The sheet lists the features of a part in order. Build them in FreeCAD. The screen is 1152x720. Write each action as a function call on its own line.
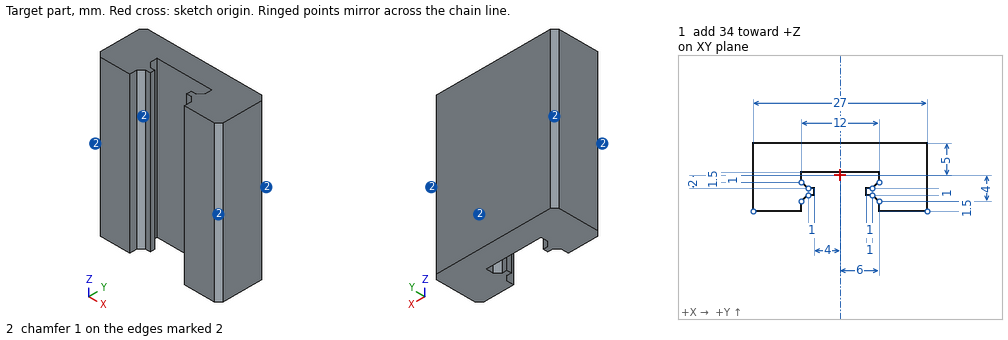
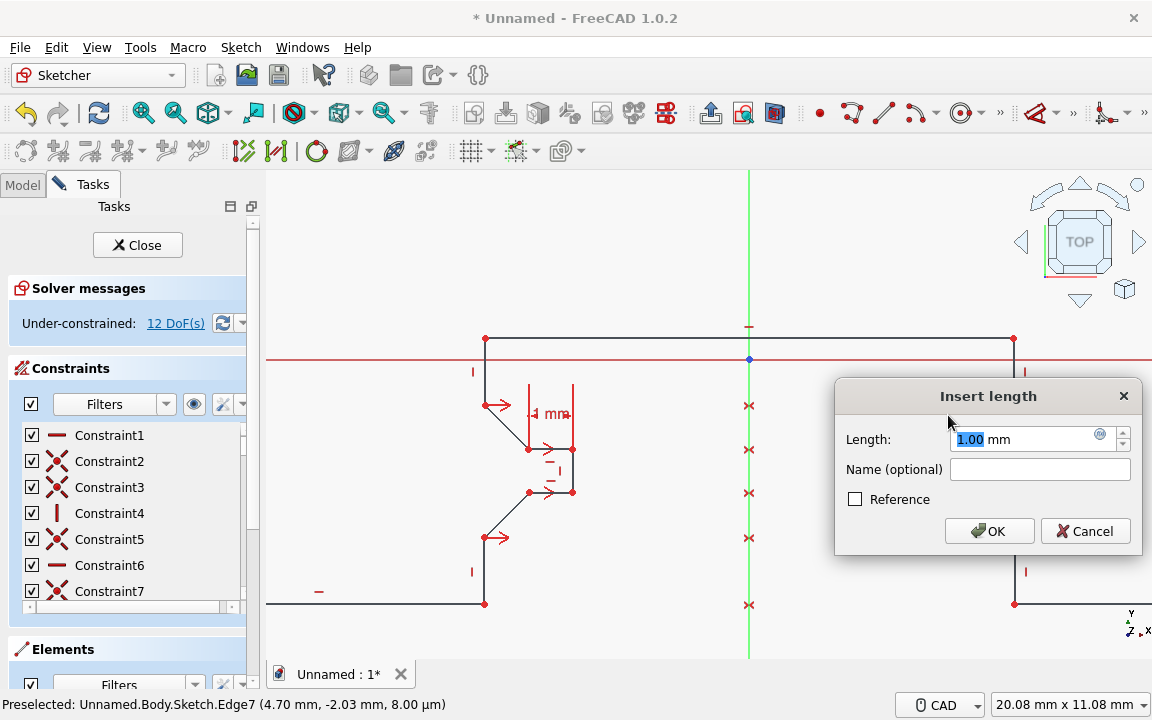
text(1)
key(Return)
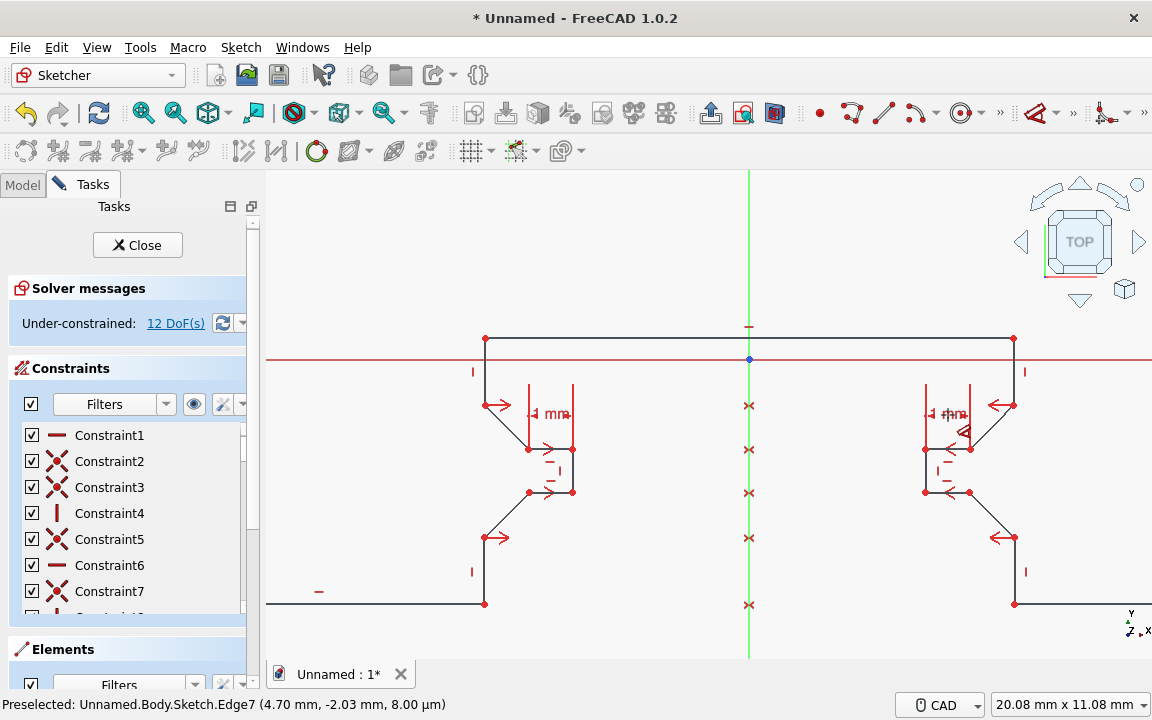
click(926, 462)
click(960, 471)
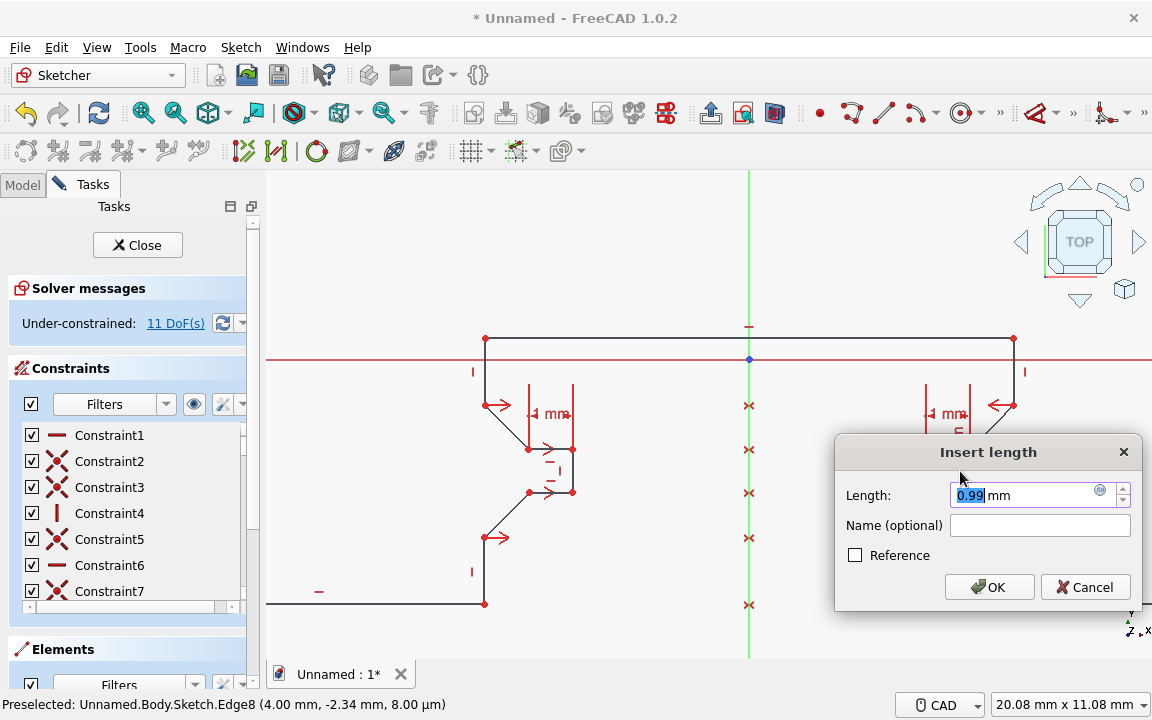
text(1)
key(Return)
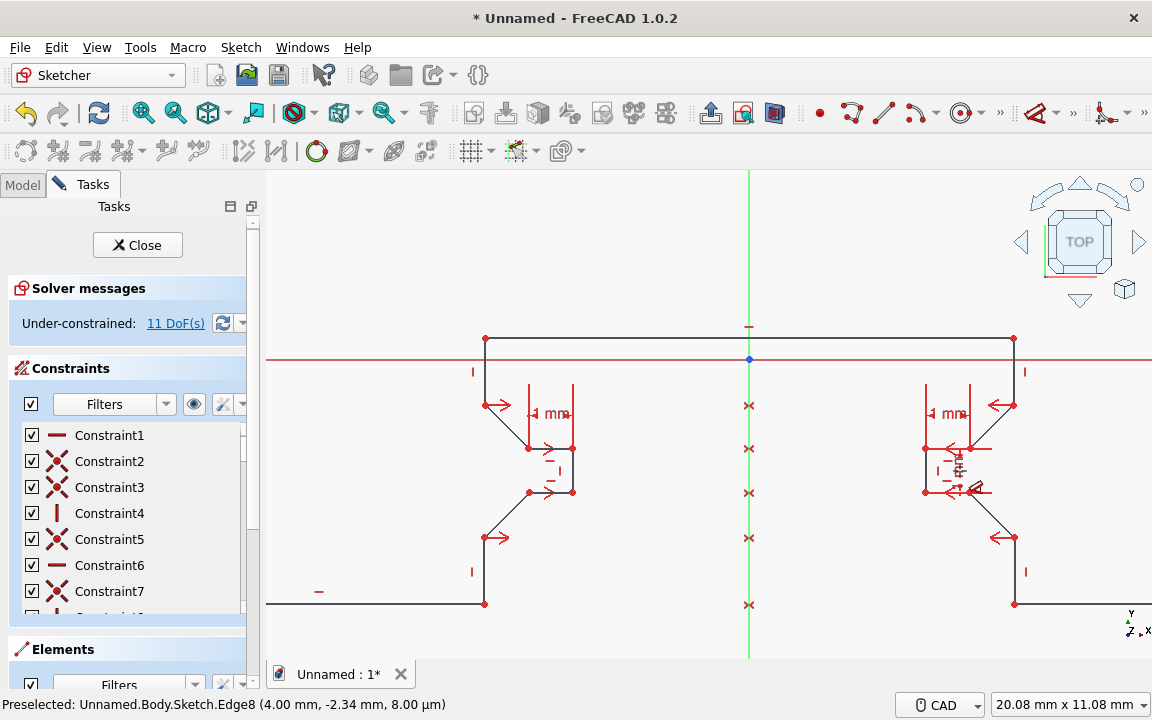
click(939, 493)
click(948, 527)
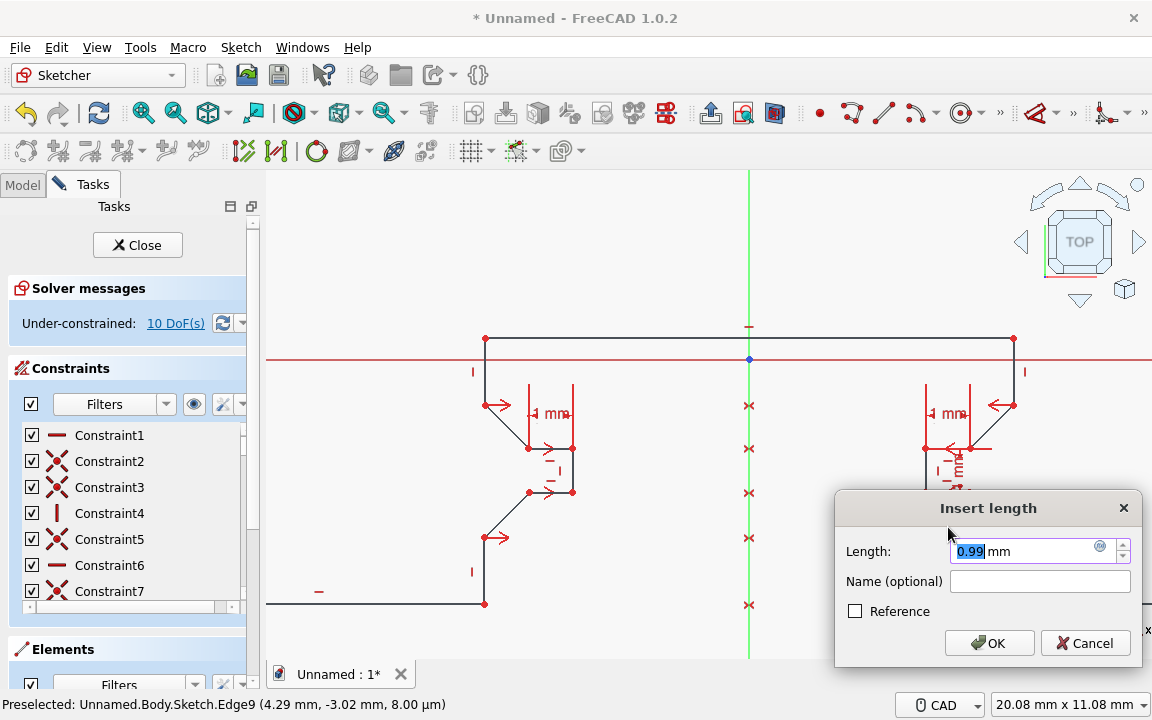
text(1)
key(Return)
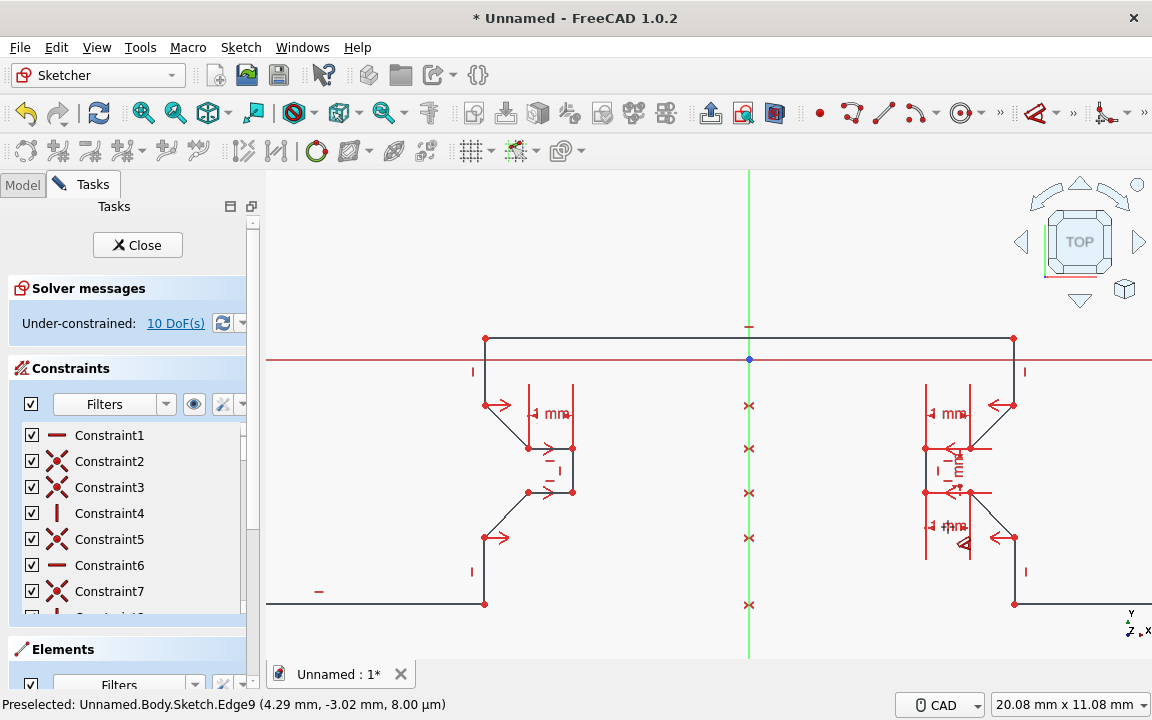
click(644, 338)
click(736, 304)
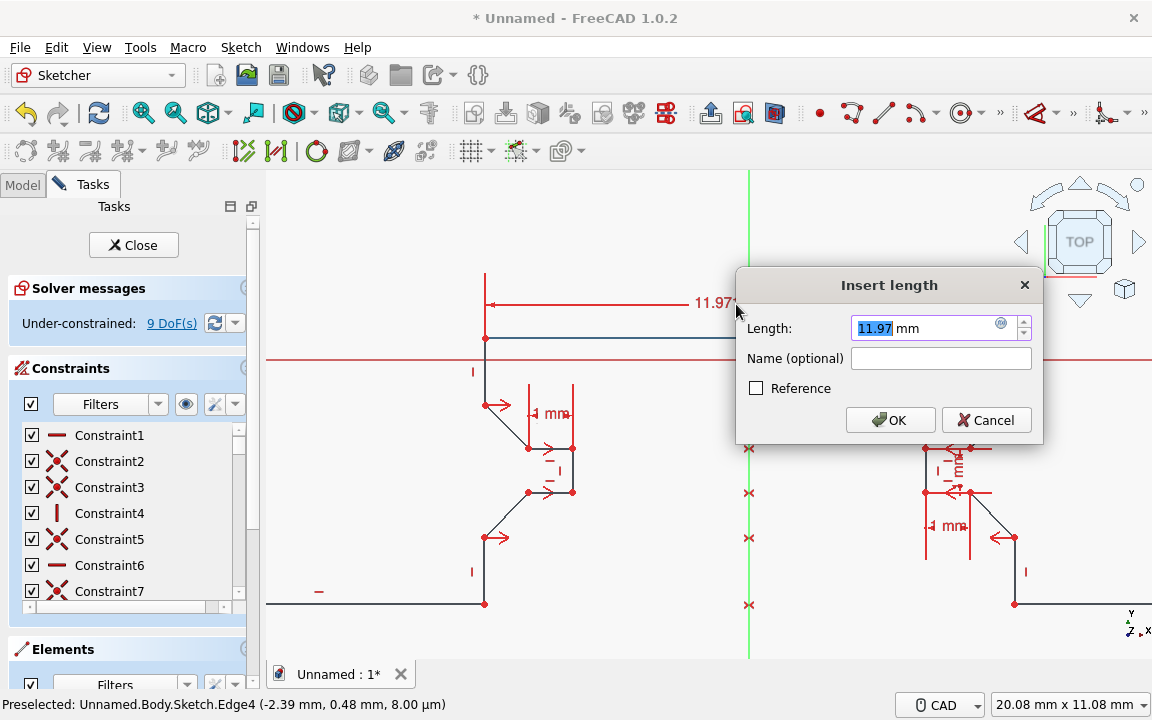
text(12)
key(Return)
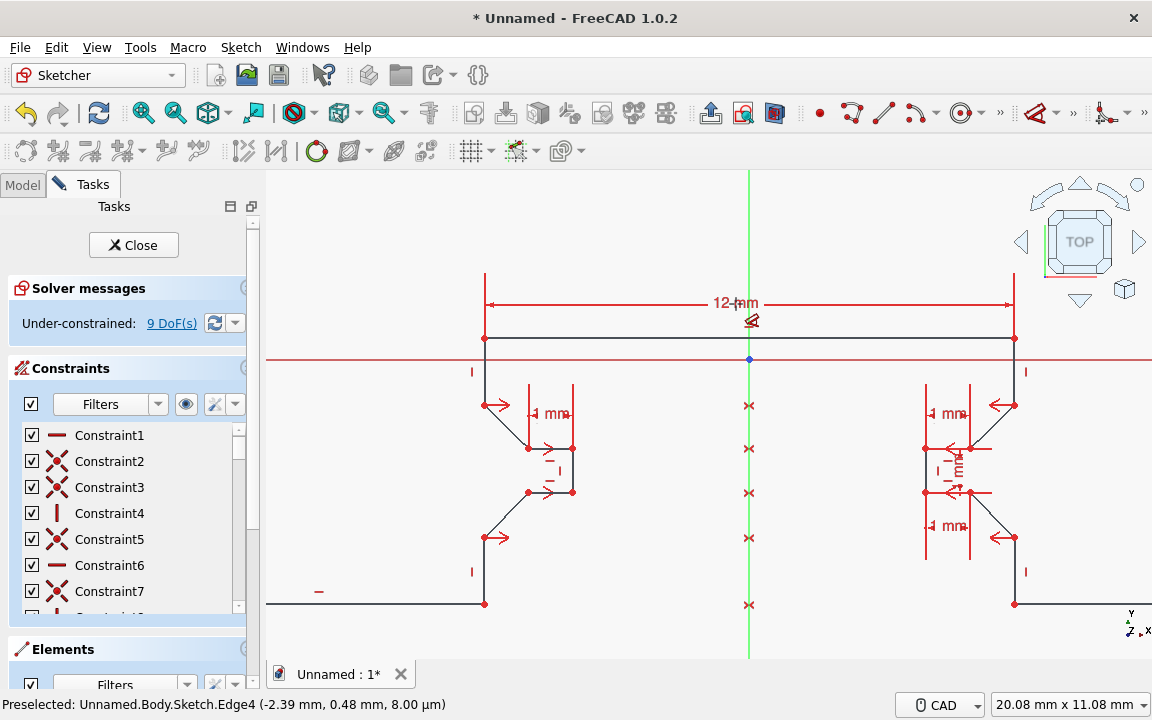
scroll(552, 450, down, 4)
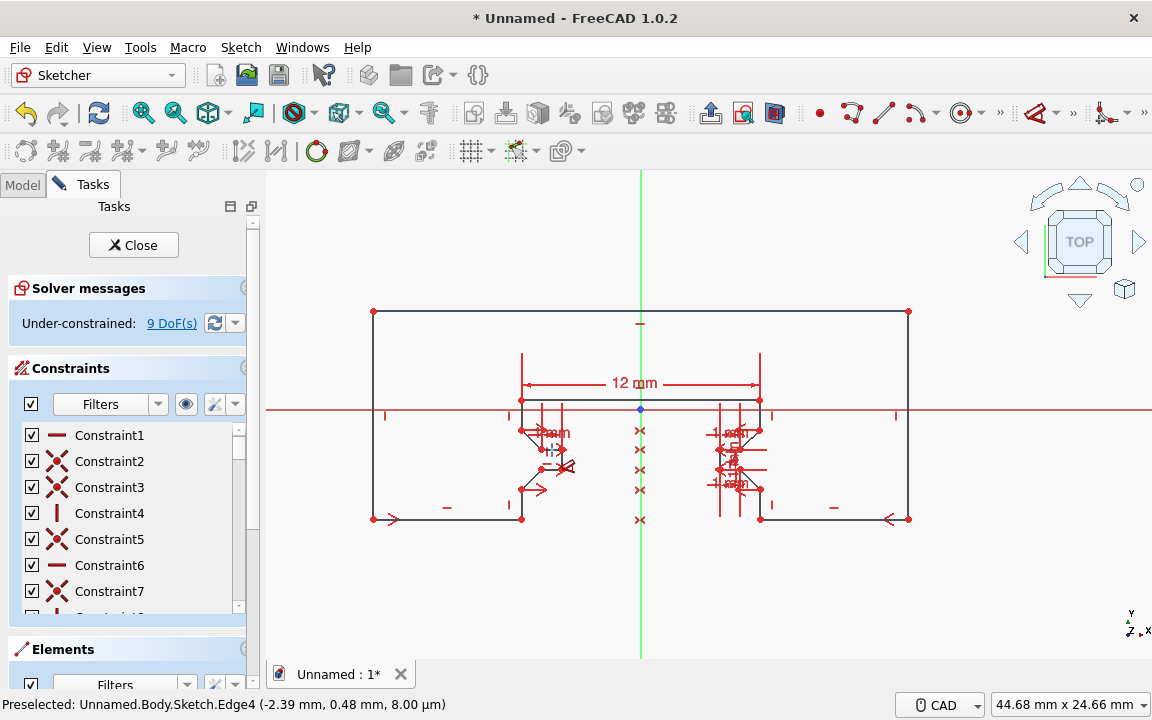
click(748, 311)
click(518, 277)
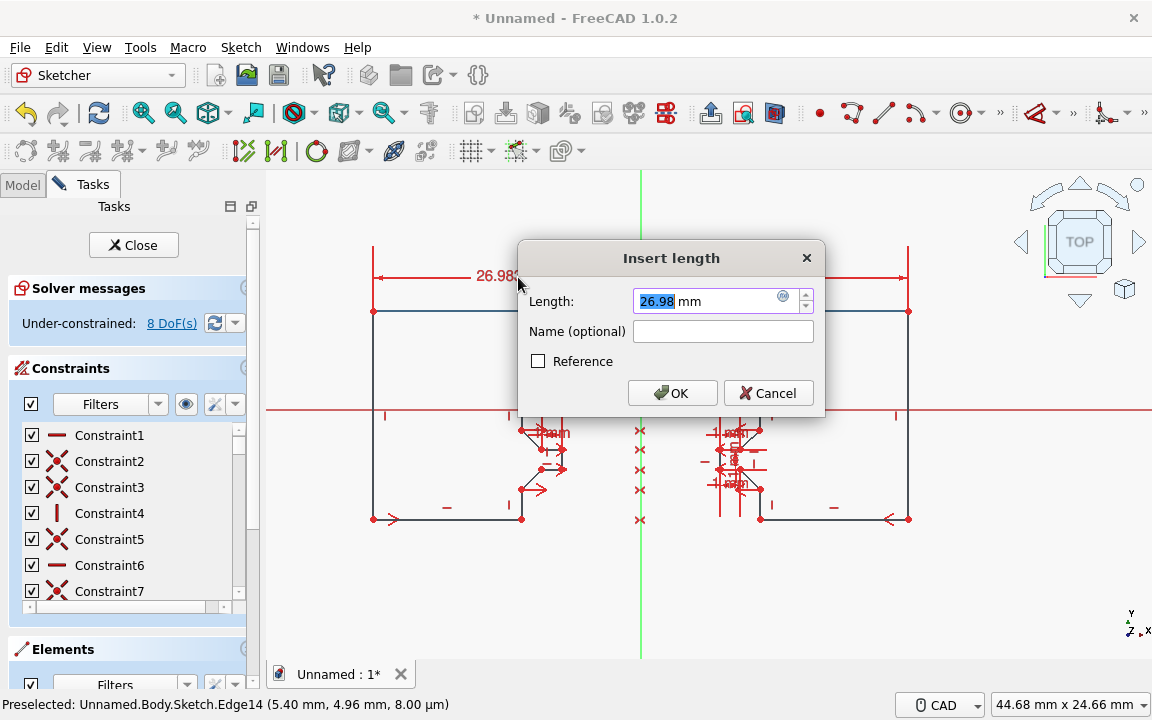
text(27)
key(Return)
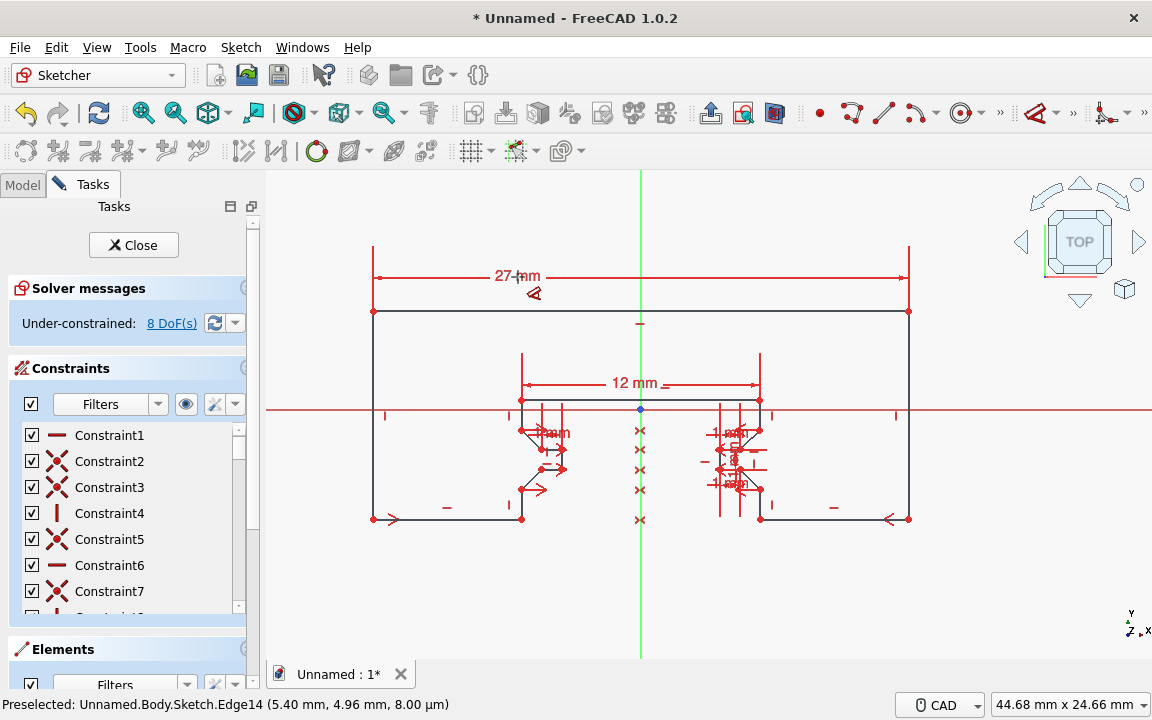
click(562, 450)
click(601, 484)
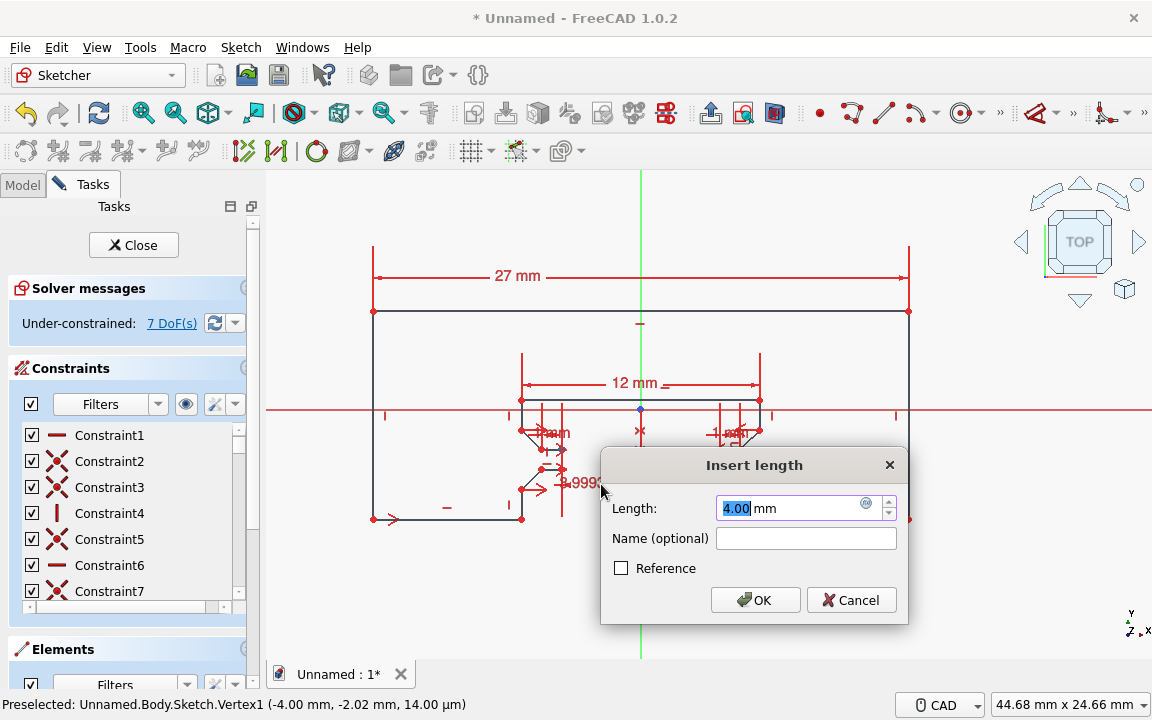
text(4)
key(Return)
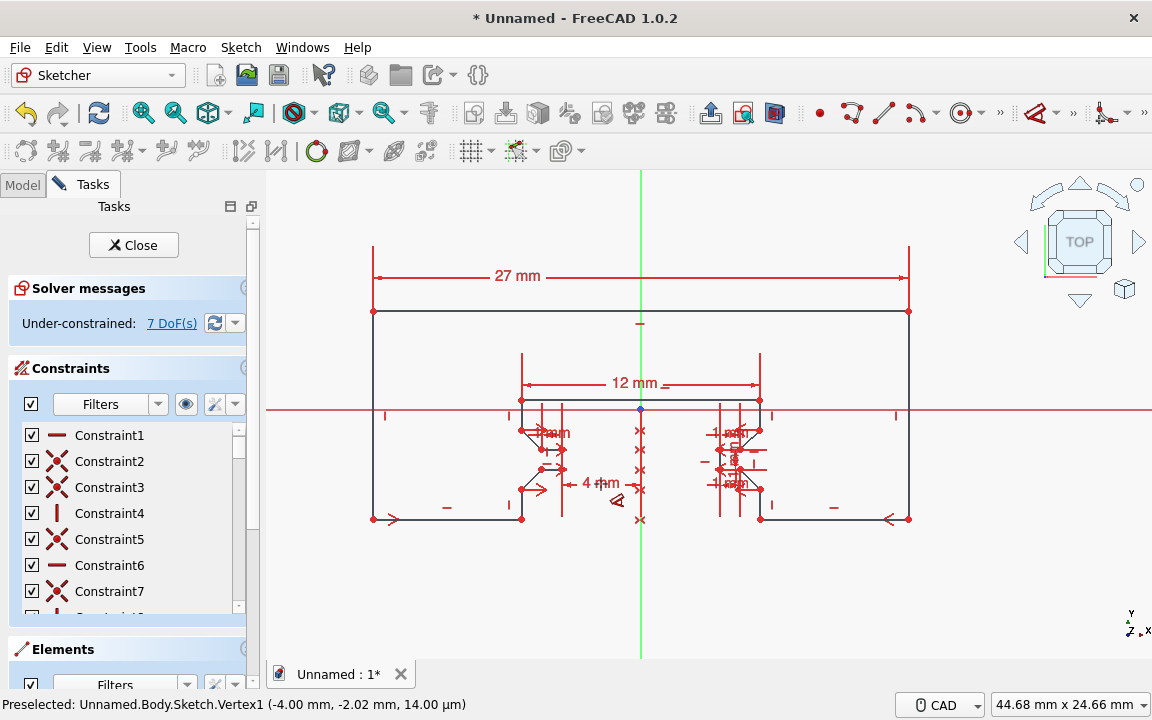
click(562, 450)
click(480, 430)